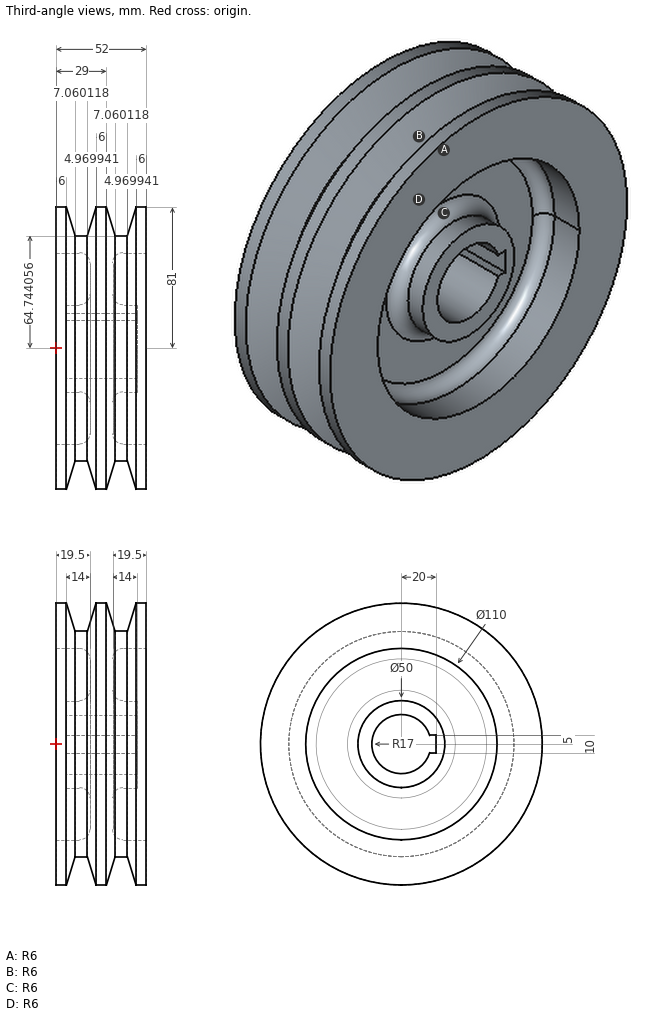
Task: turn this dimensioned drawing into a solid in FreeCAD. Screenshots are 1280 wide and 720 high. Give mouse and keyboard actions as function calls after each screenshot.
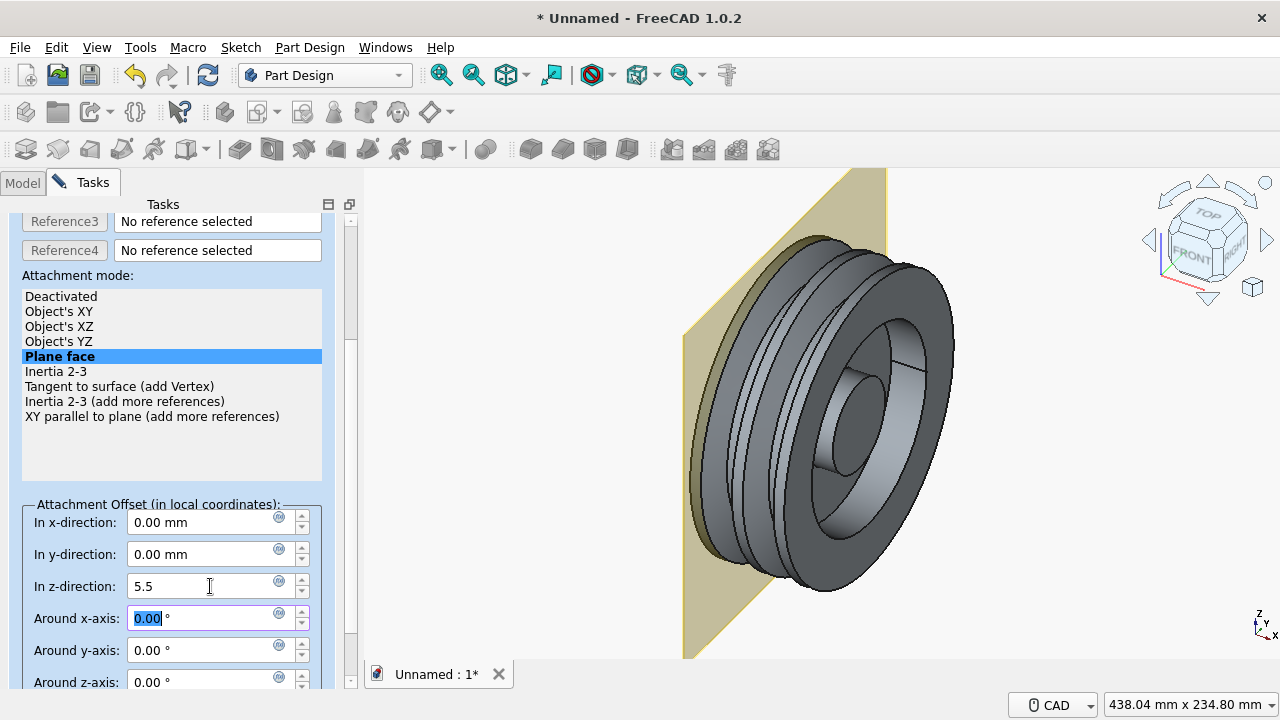
scroll(351, 451, up, 4)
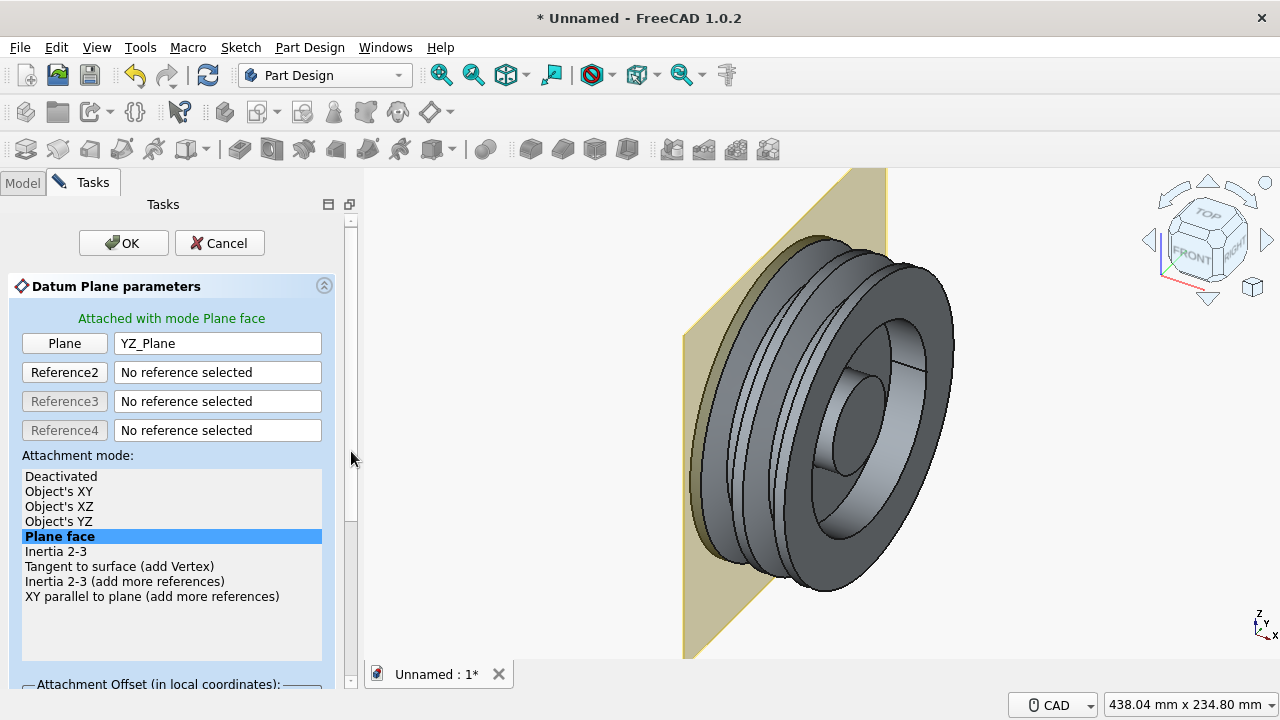
click(124, 243)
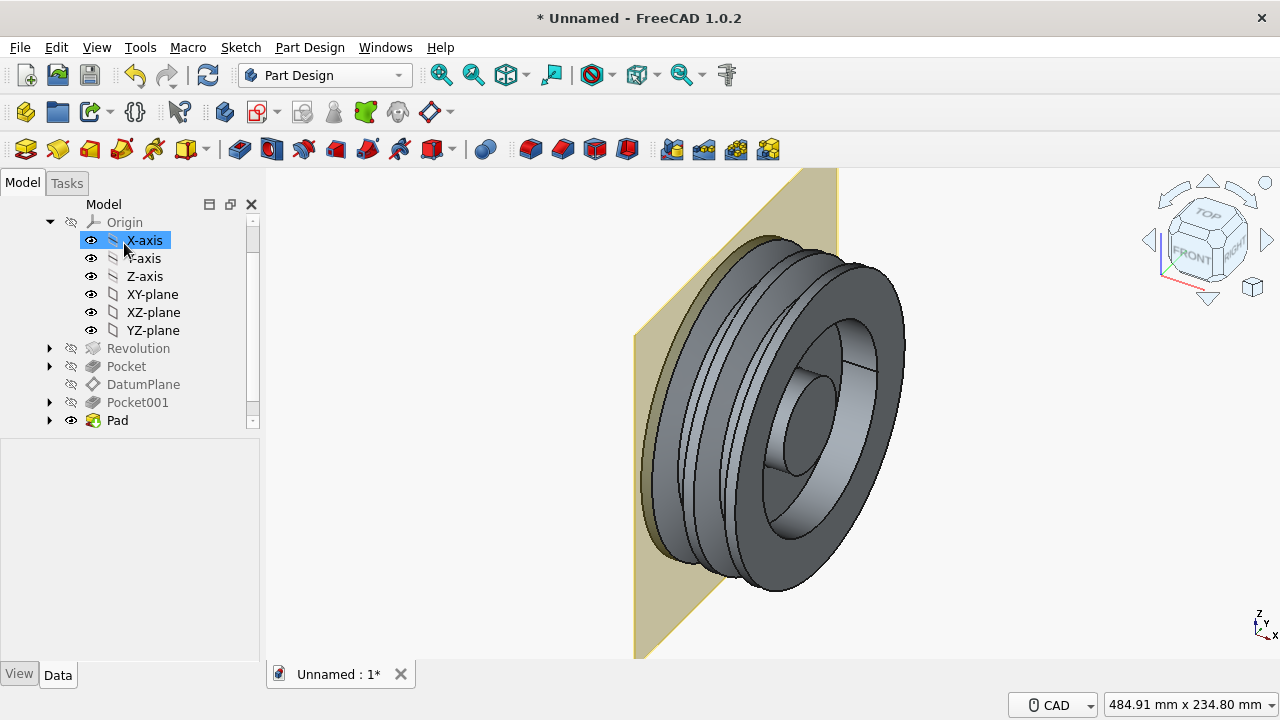
scroll(140, 326, down, 3)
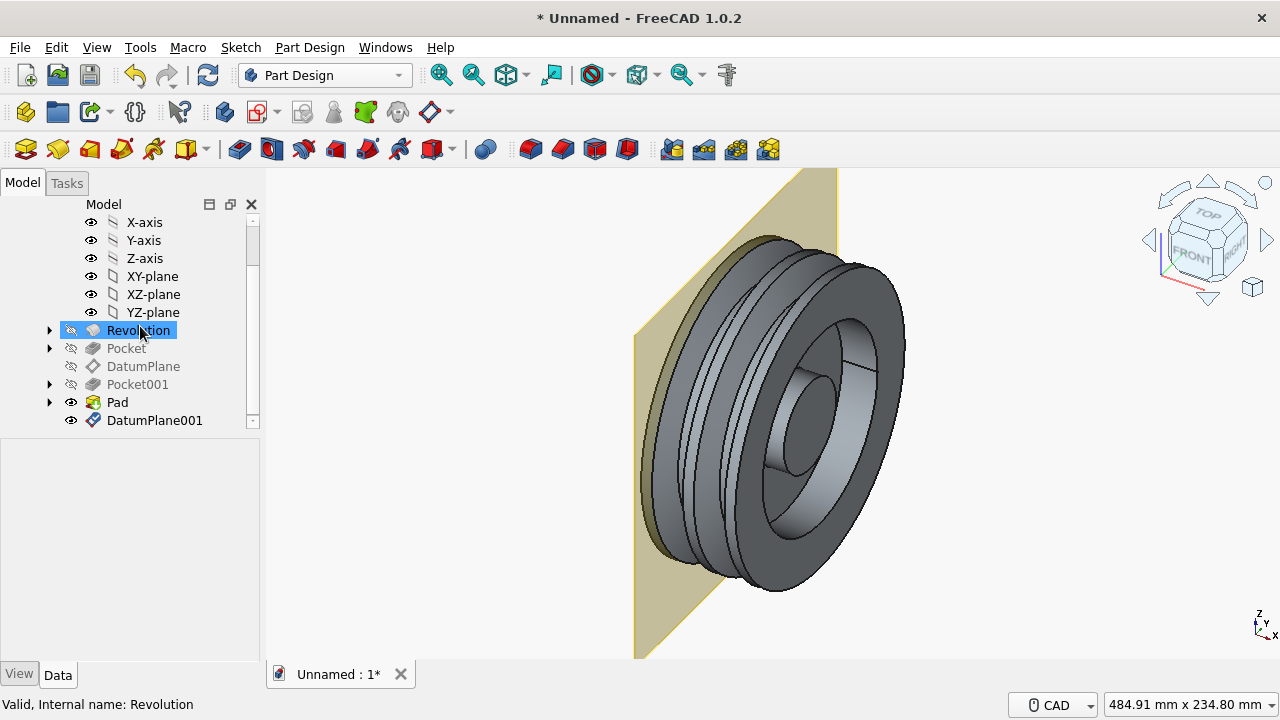
click(116, 420)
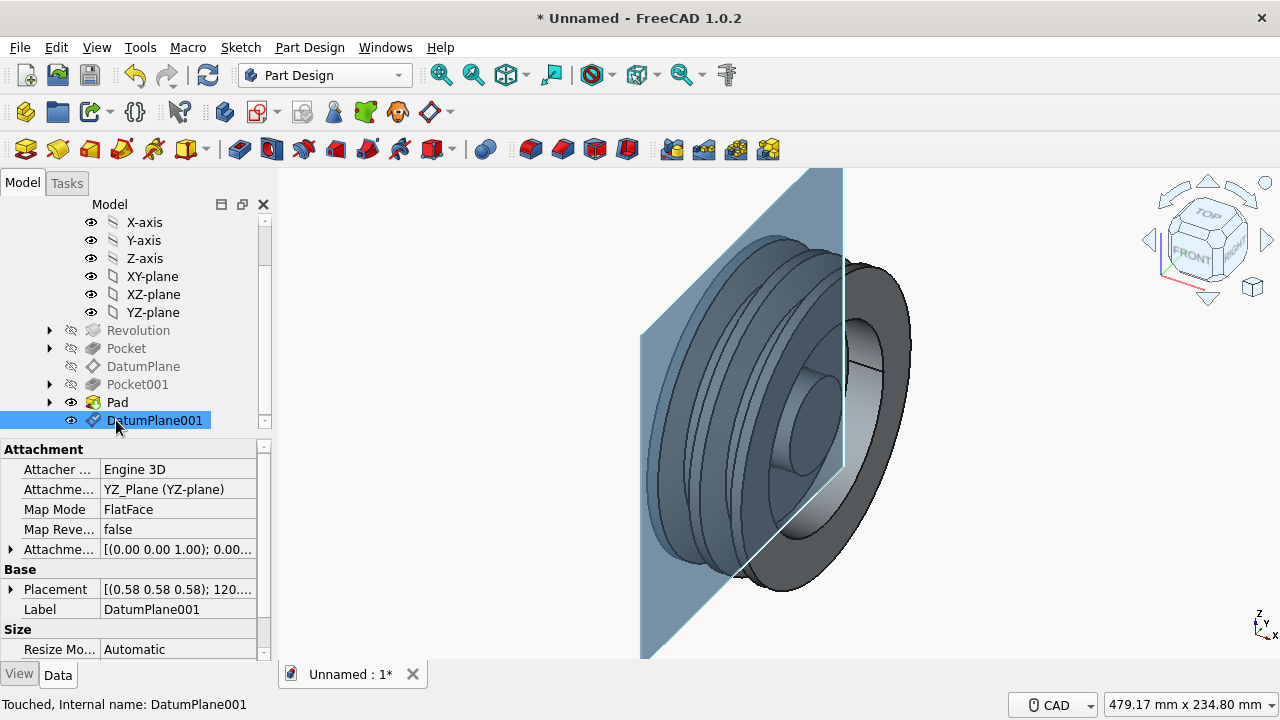
click(258, 112)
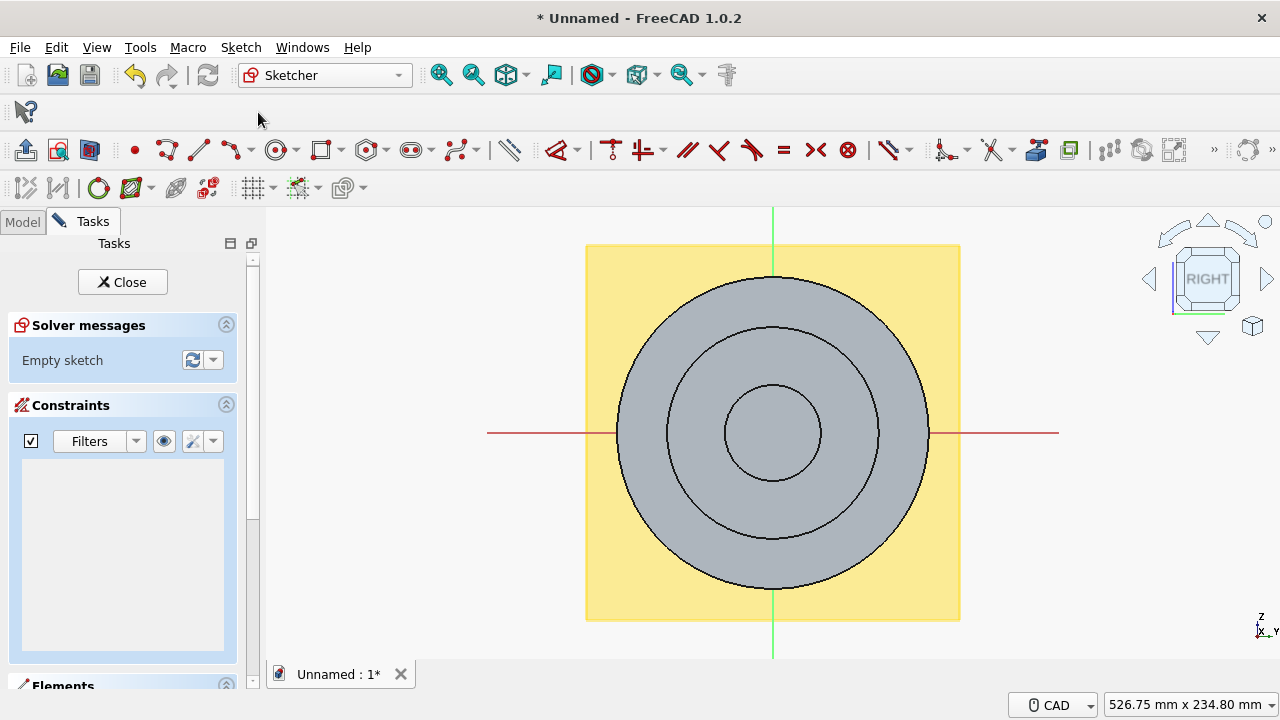
key(q)
key(s)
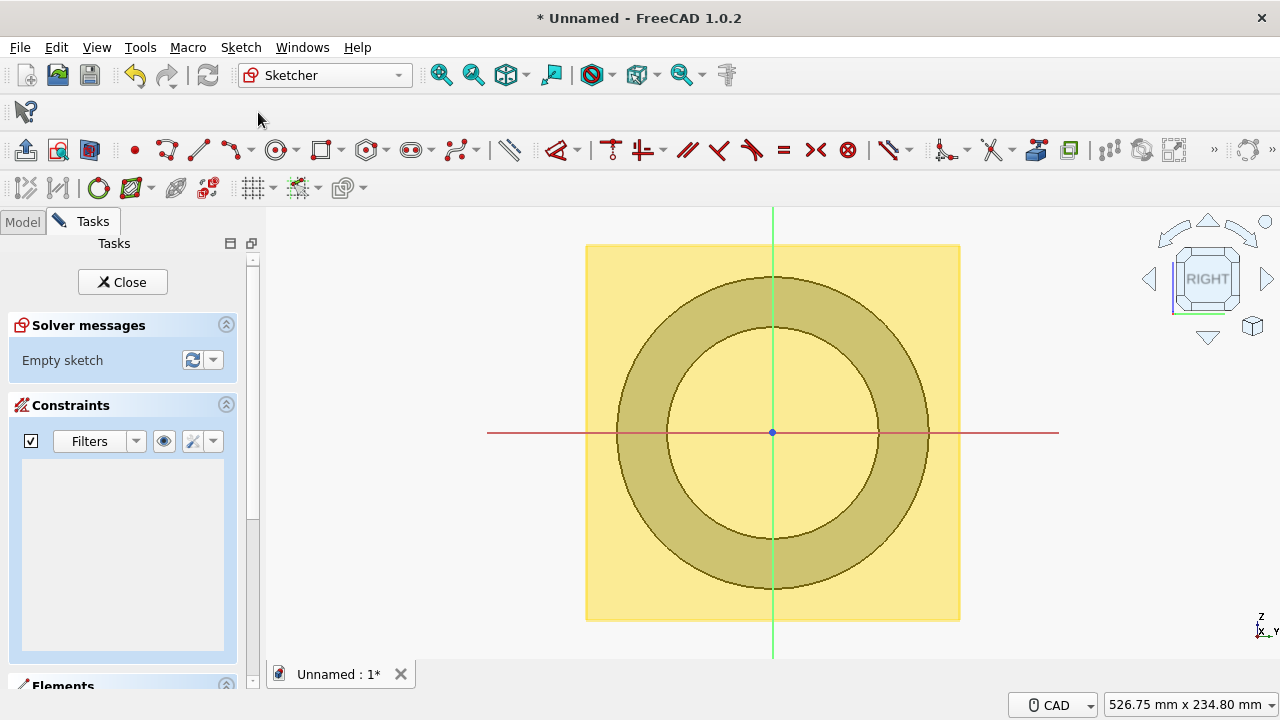
scroll(813, 433, up, 5)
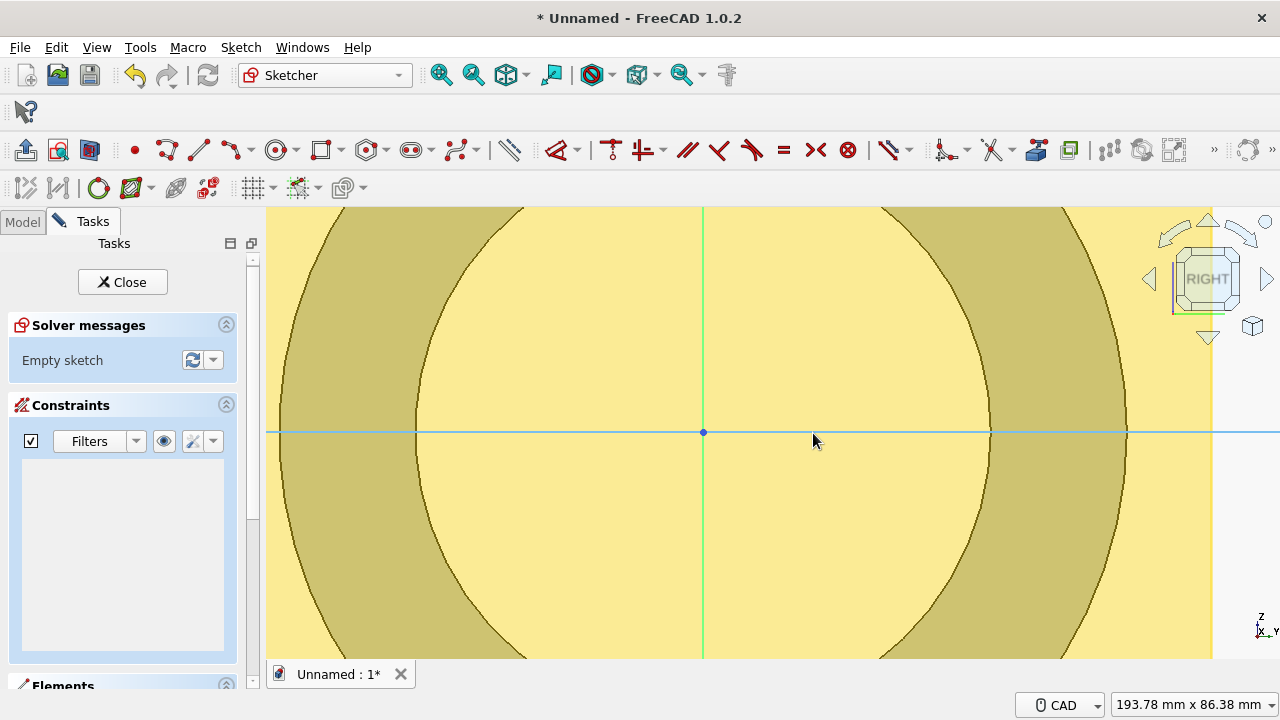
key(g)
key(c)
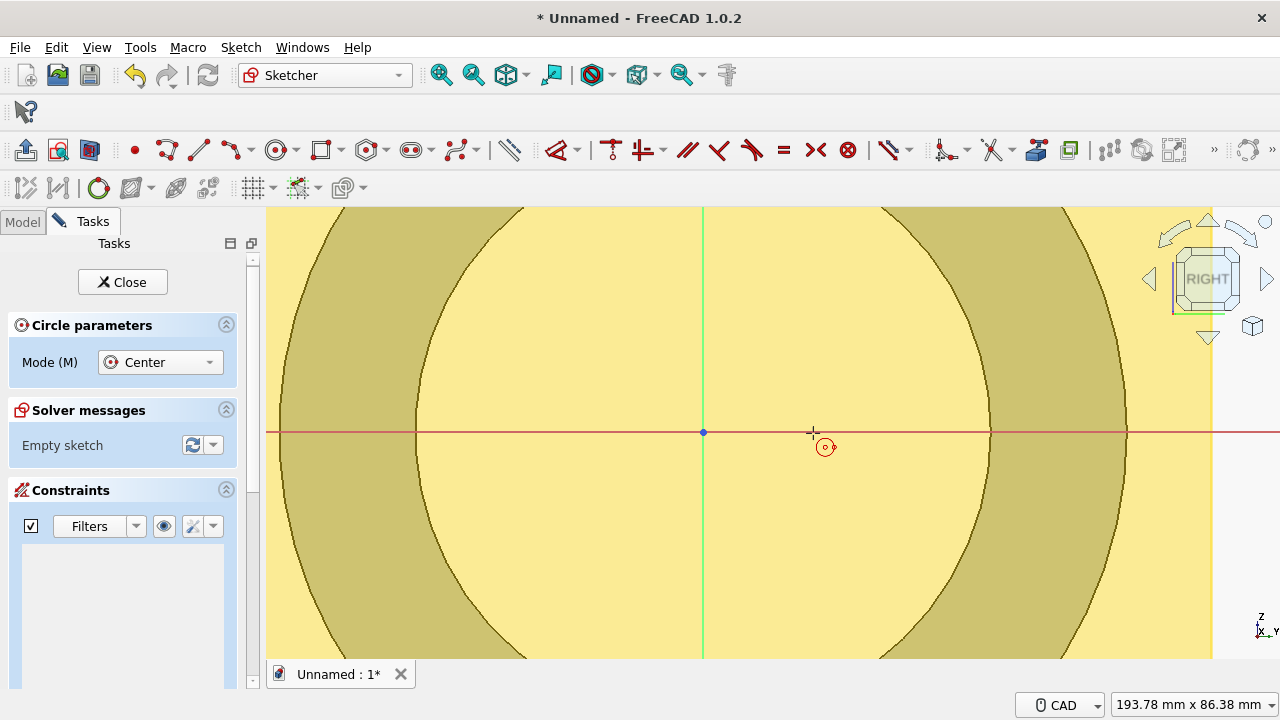
click(703, 432)
click(796, 340)
key(Escape)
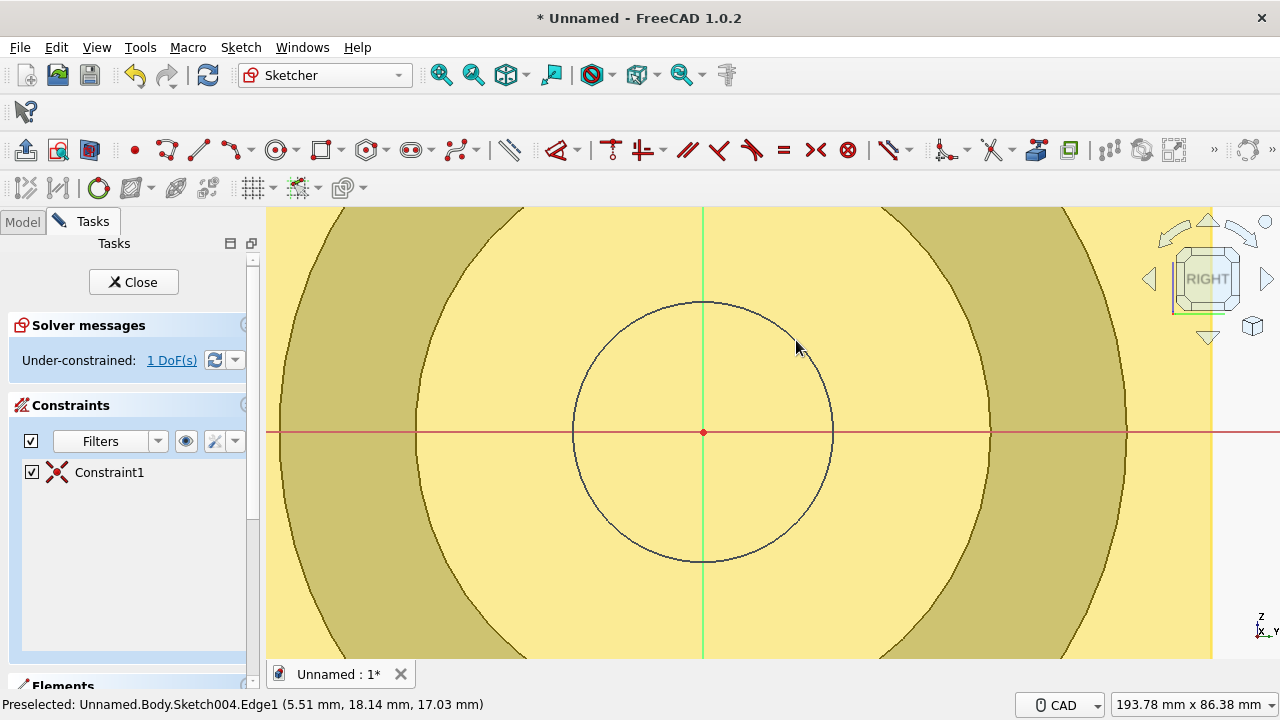
key(d)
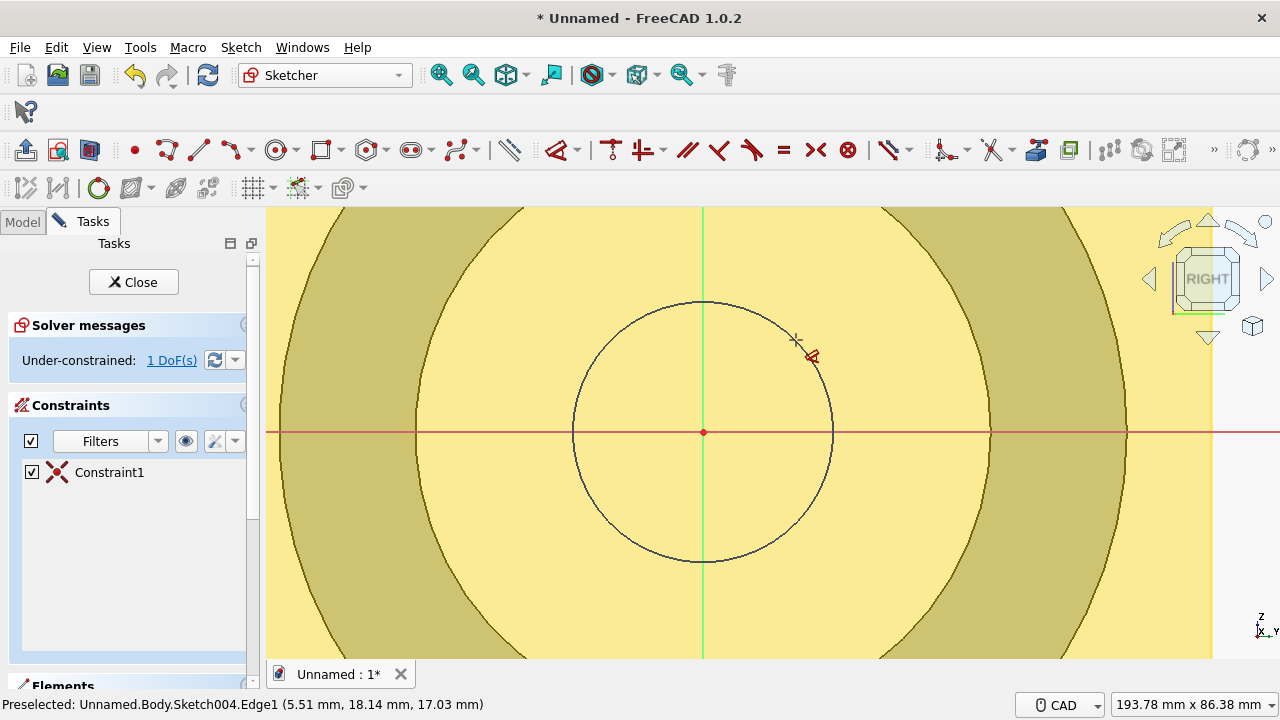
click(795, 340)
click(818, 317)